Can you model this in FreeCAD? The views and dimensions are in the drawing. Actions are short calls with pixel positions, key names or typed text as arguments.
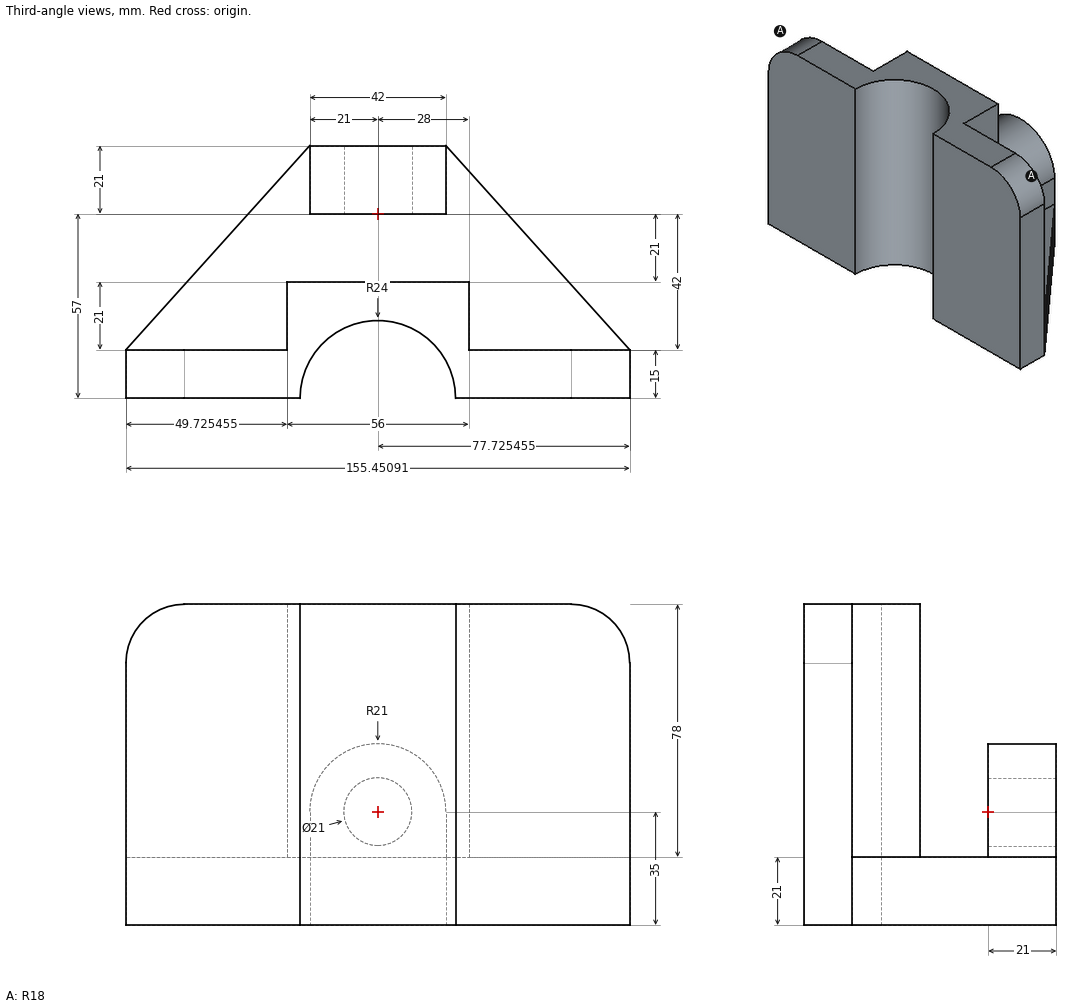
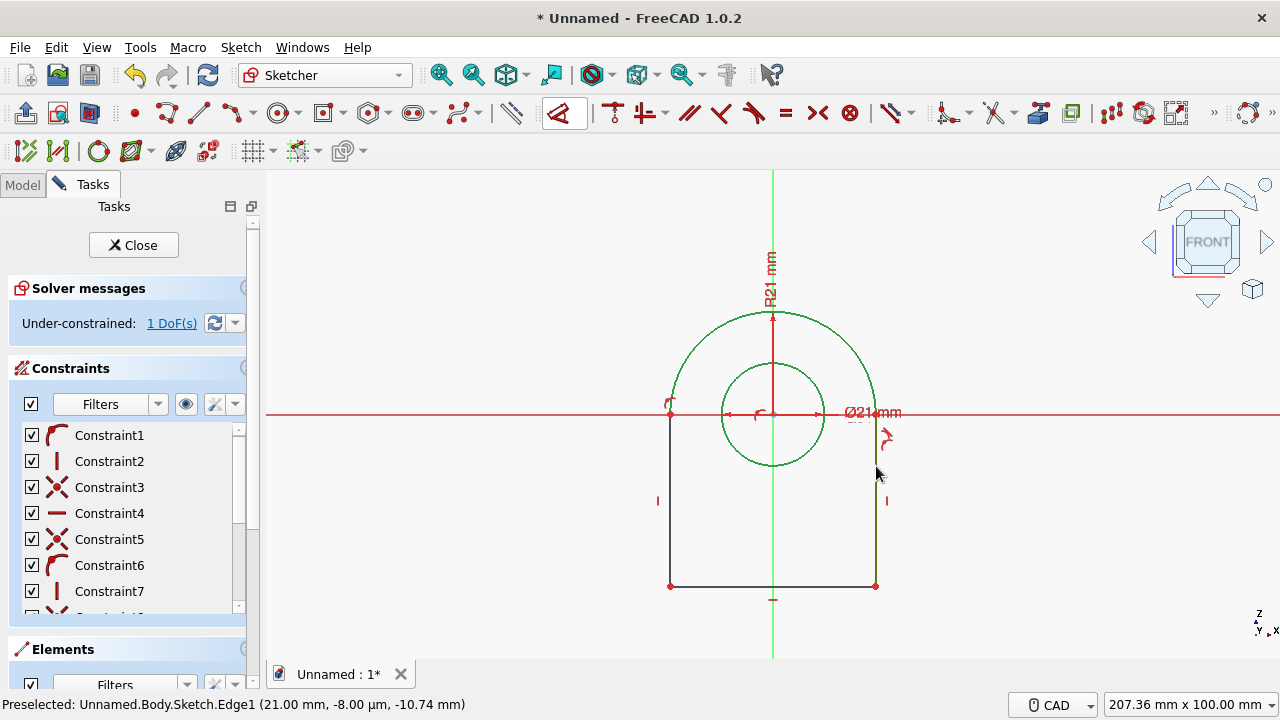
key(i)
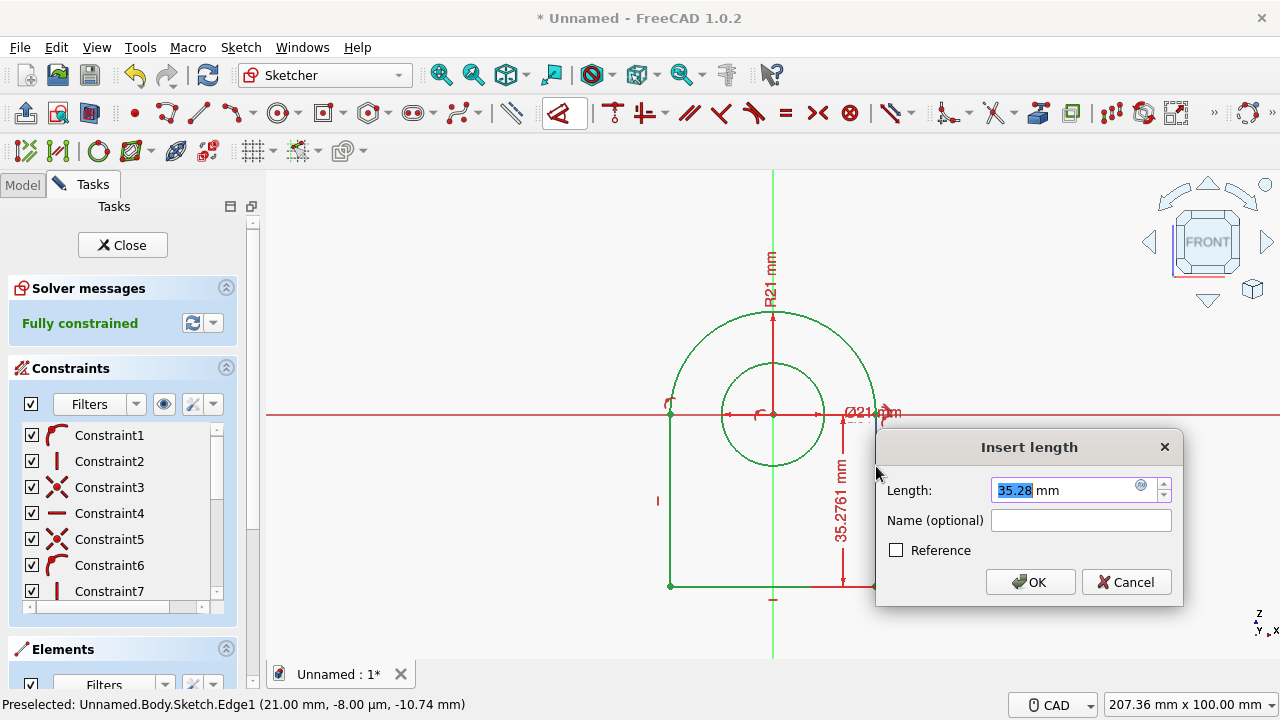
text(35)
key(Return)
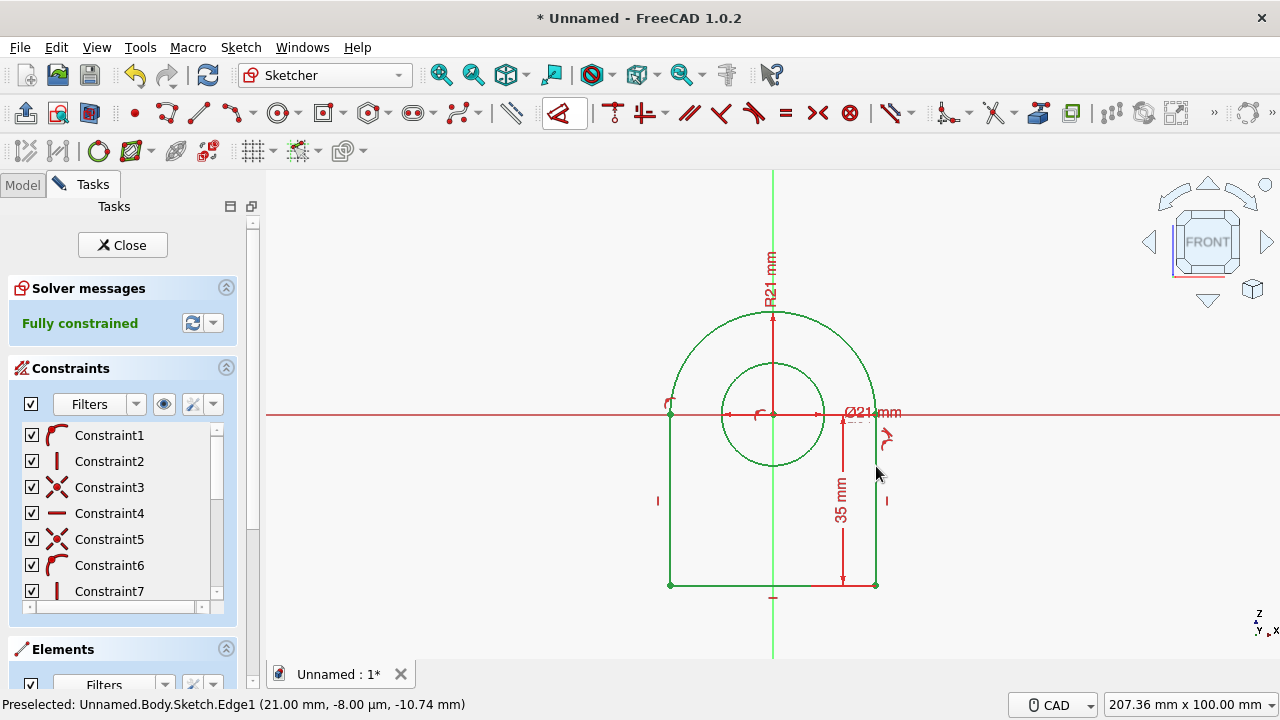
click(123, 245)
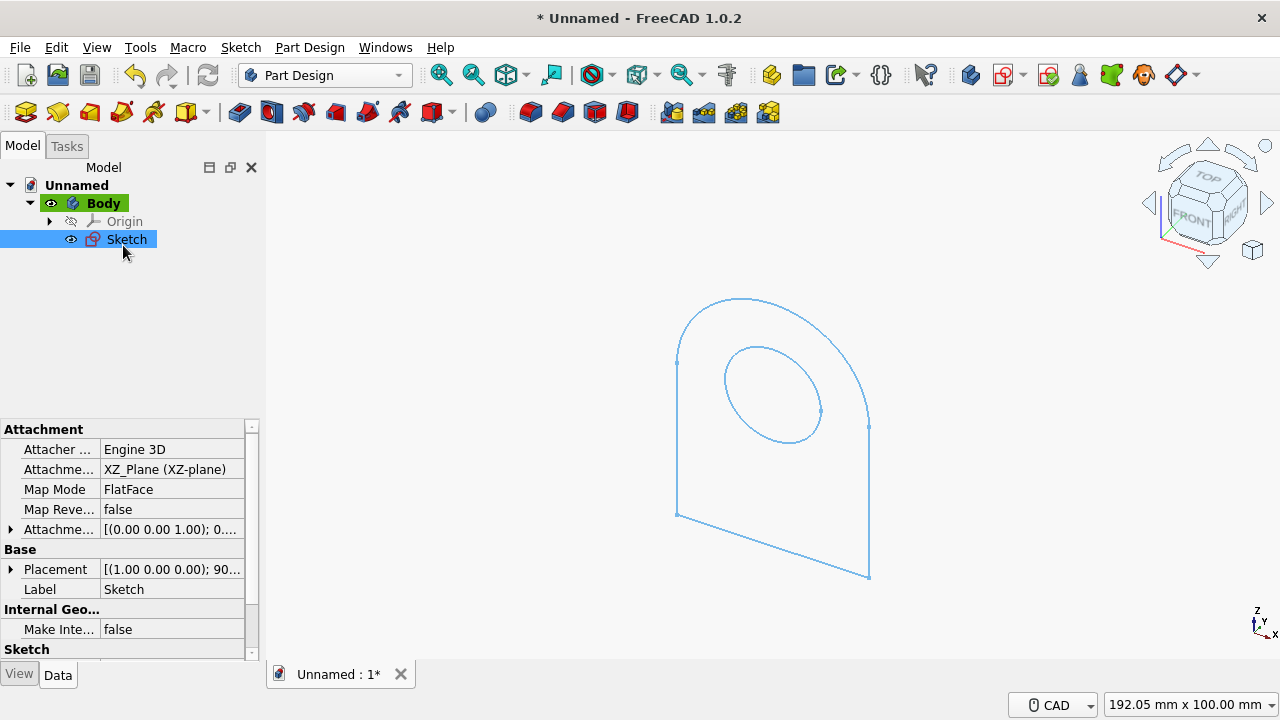
click(26, 112)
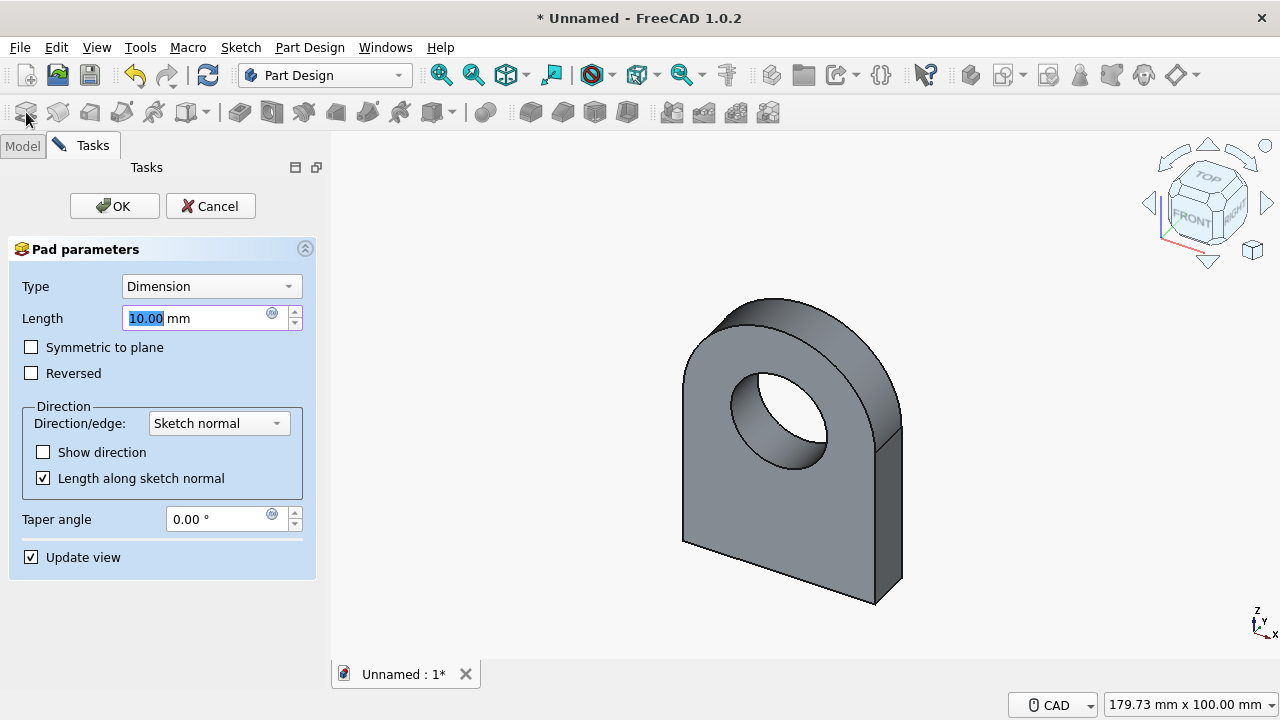
text(21)
key(Tab)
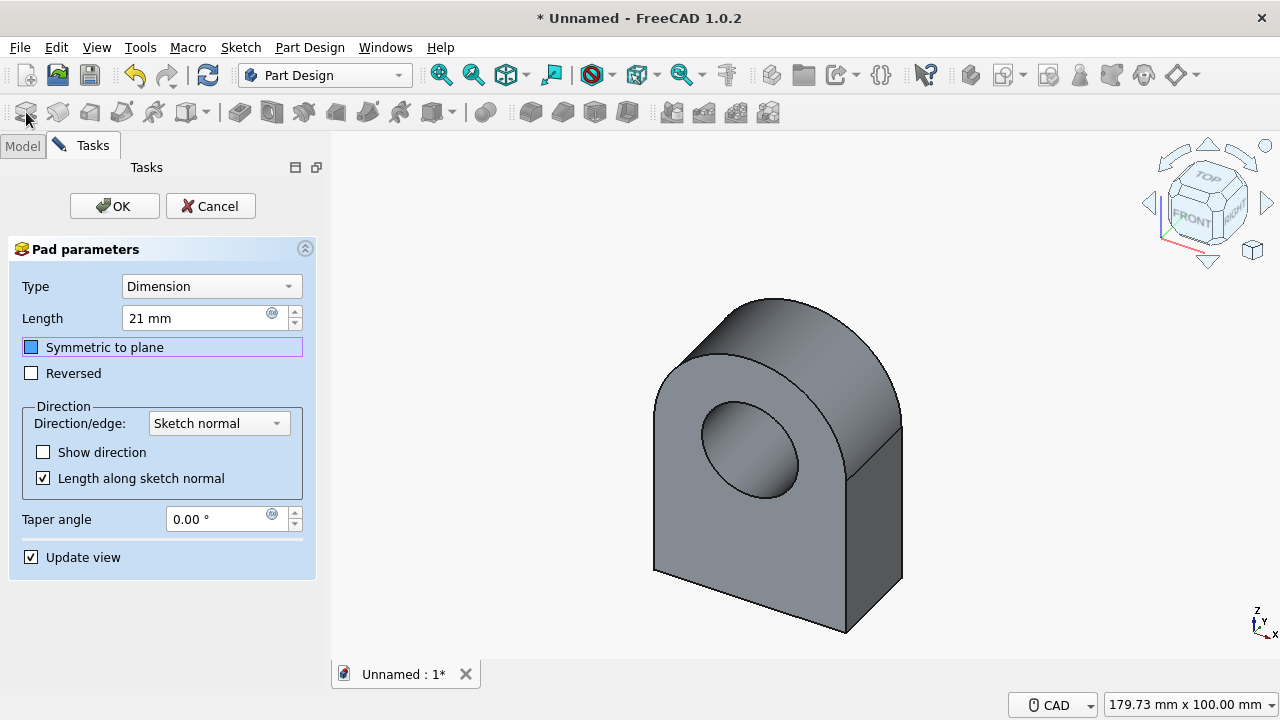
click(30, 373)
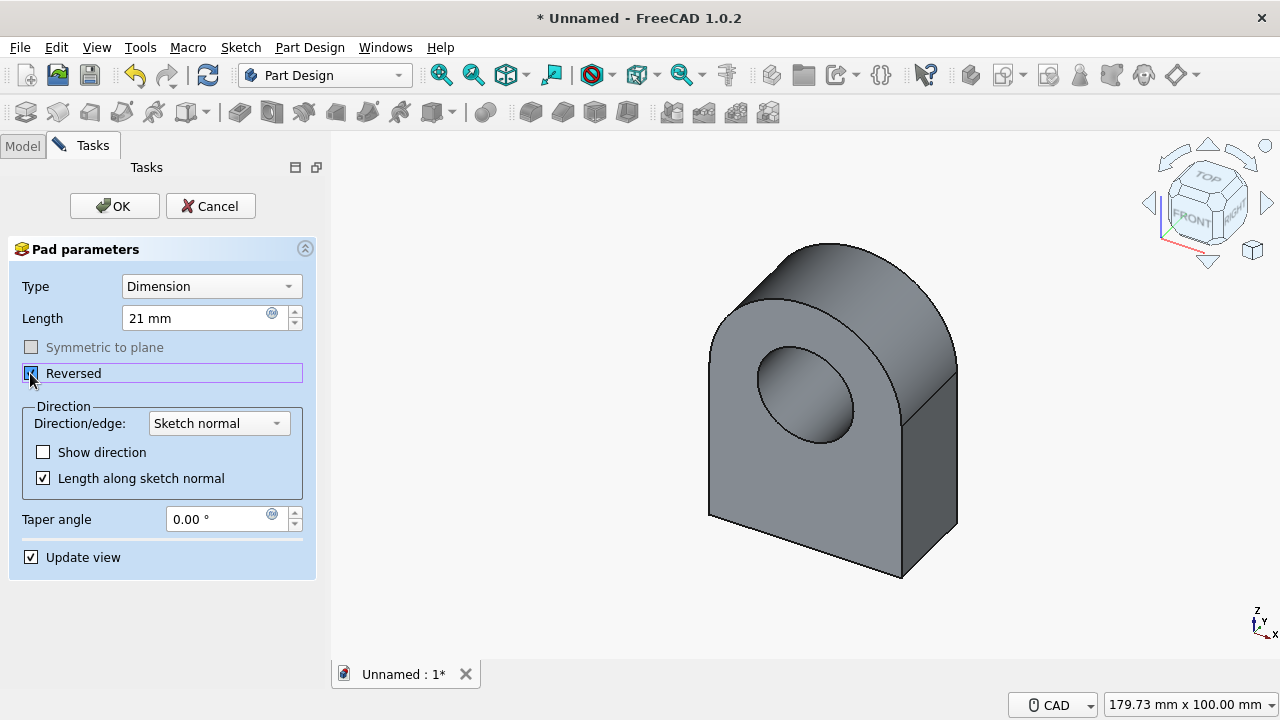
click(115, 206)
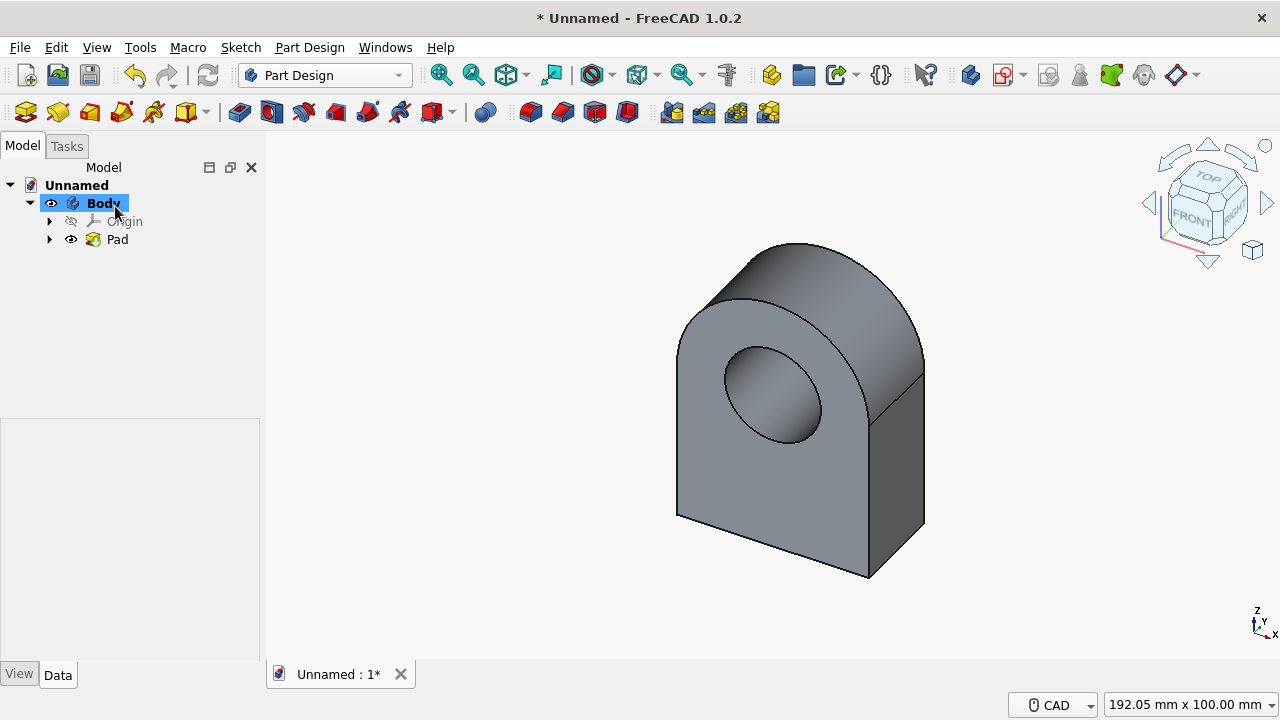
key(5)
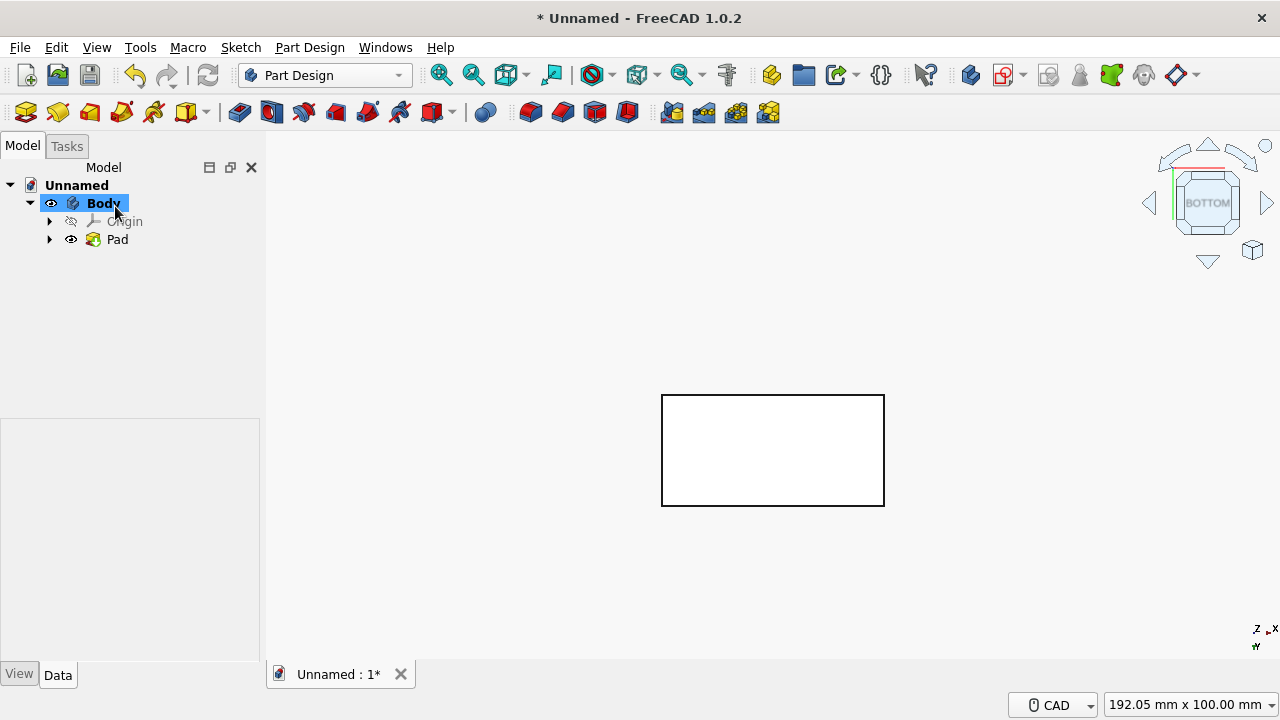
click(442, 76)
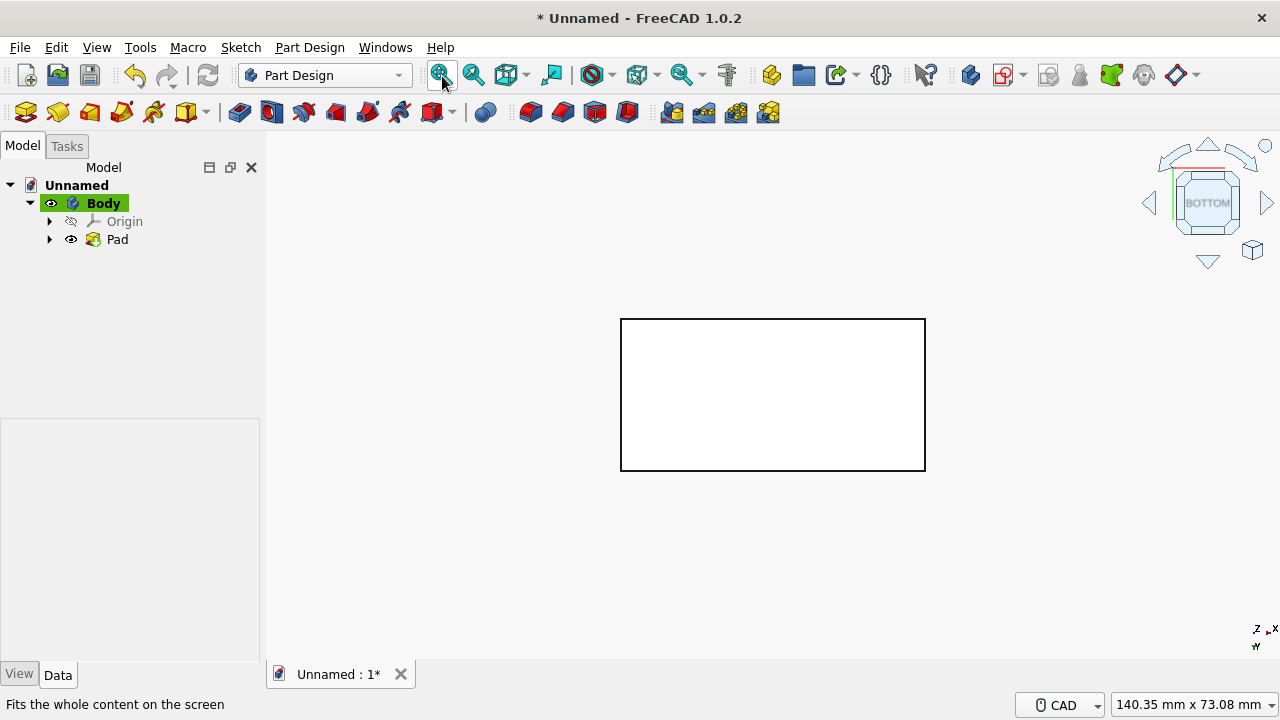
click(816, 394)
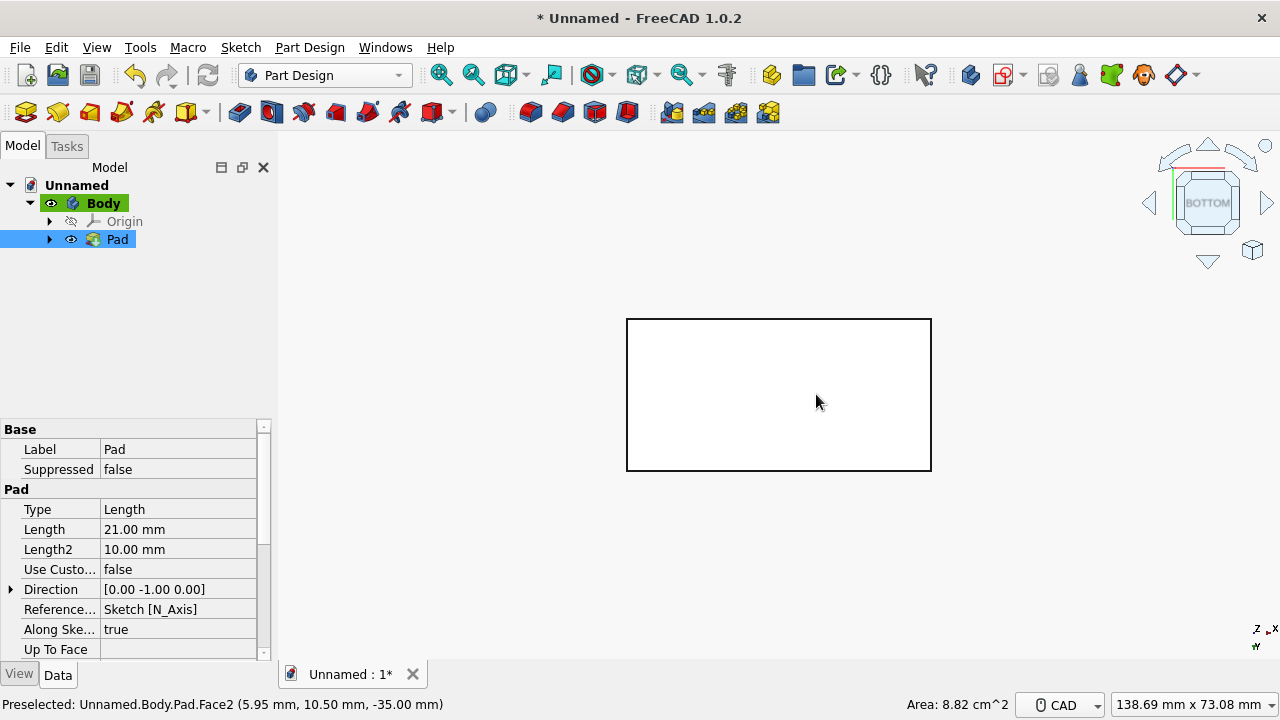
click(1004, 76)